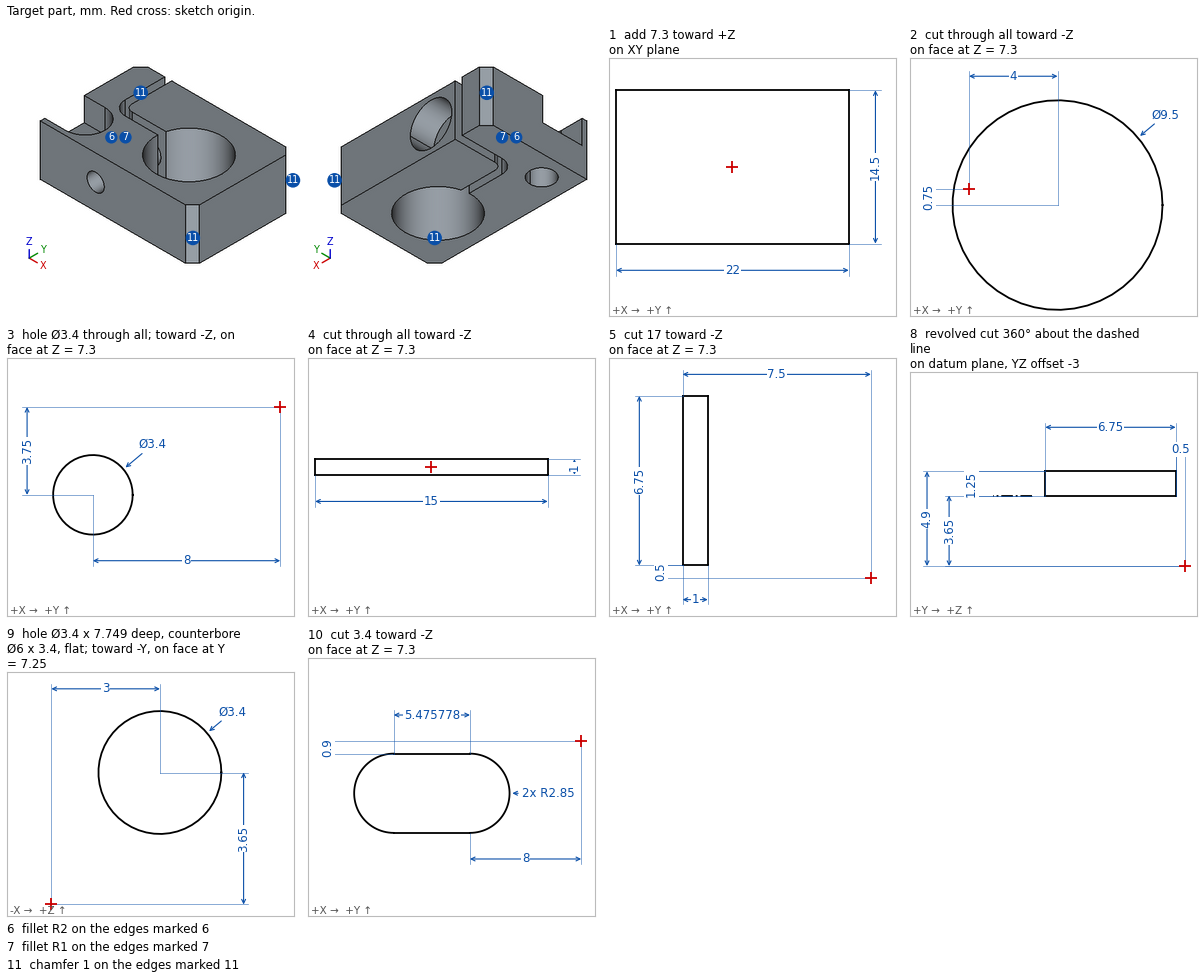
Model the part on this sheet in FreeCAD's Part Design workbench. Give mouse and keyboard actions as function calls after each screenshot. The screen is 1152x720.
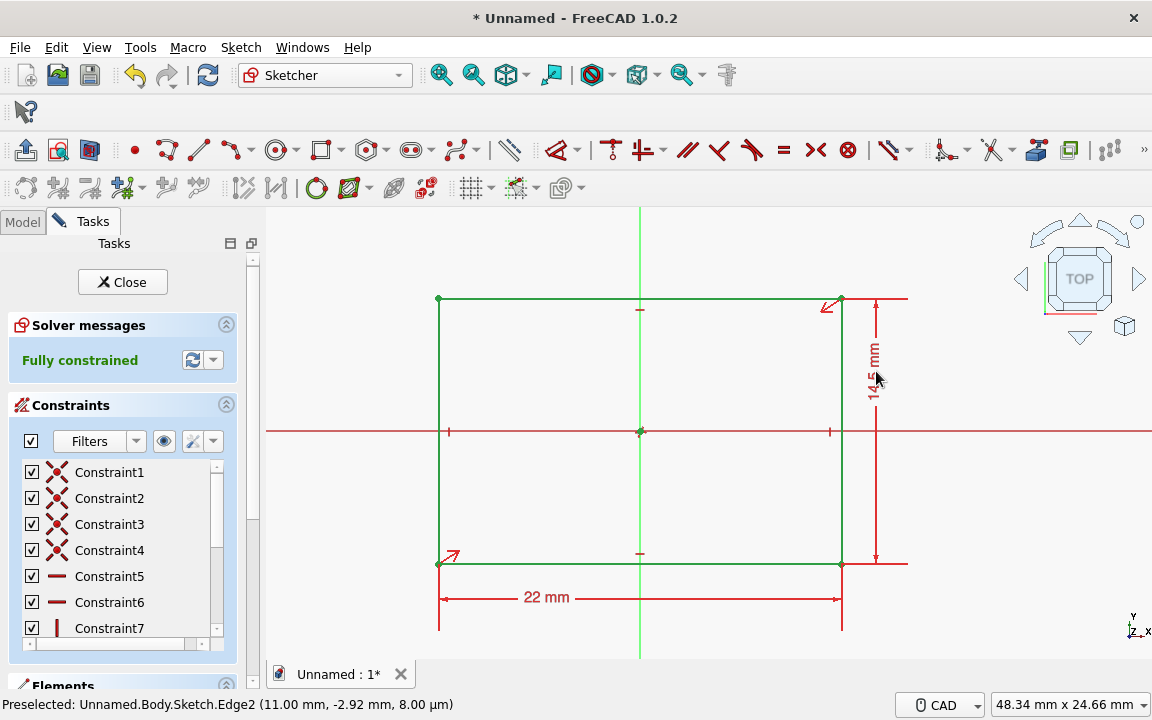
click(123, 282)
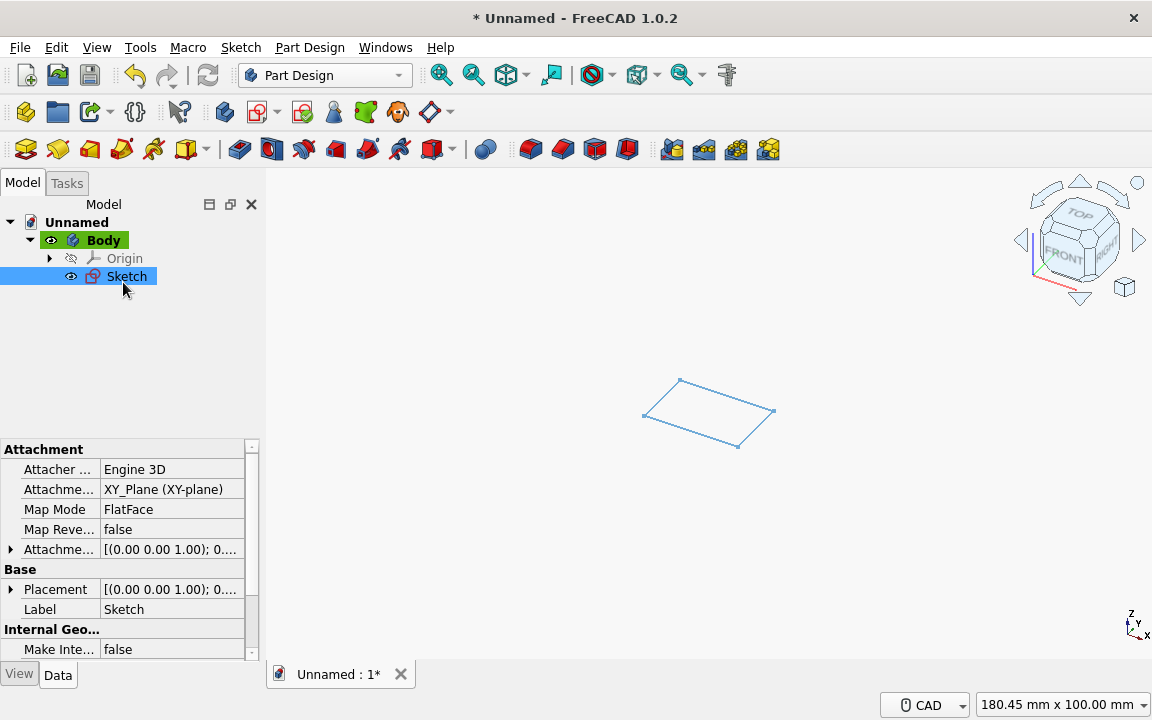
click(26, 150)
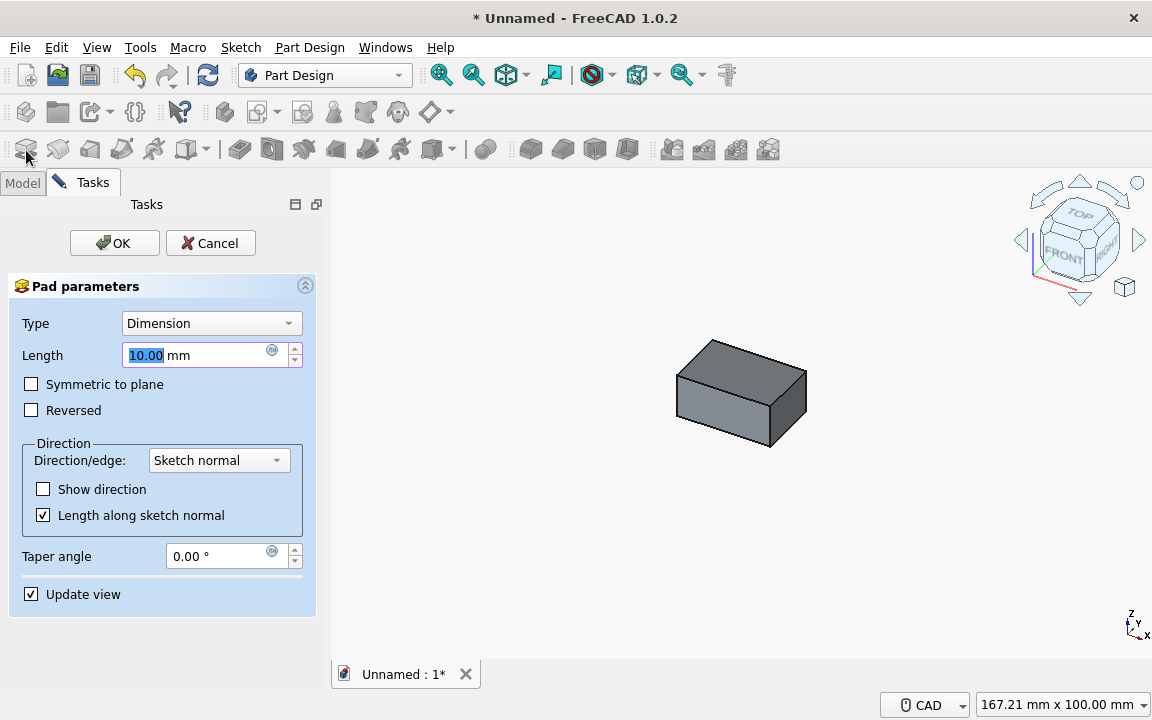
text(7.3)
key(Tab)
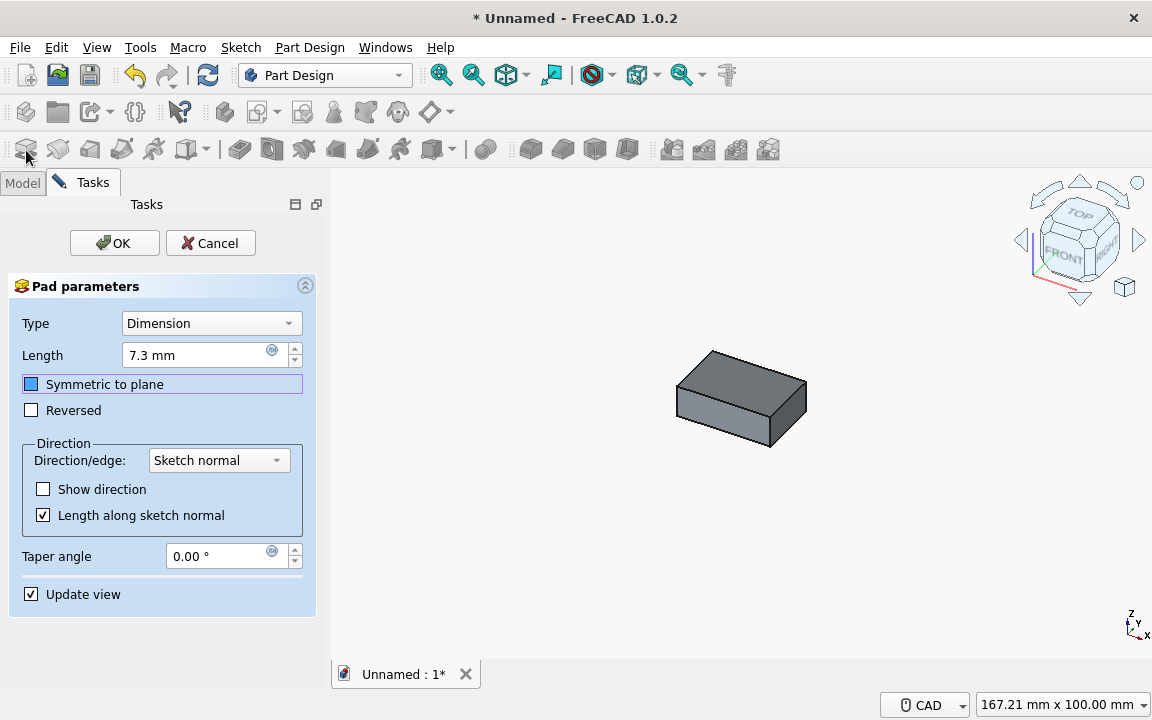
click(115, 243)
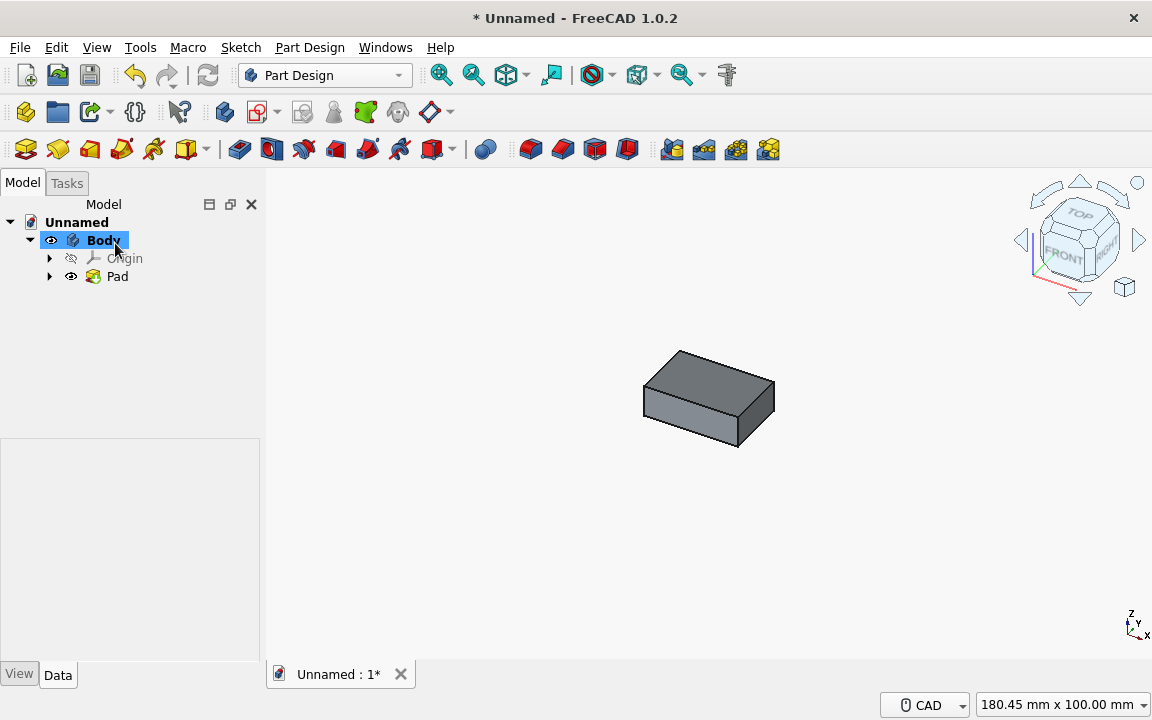
click(442, 76)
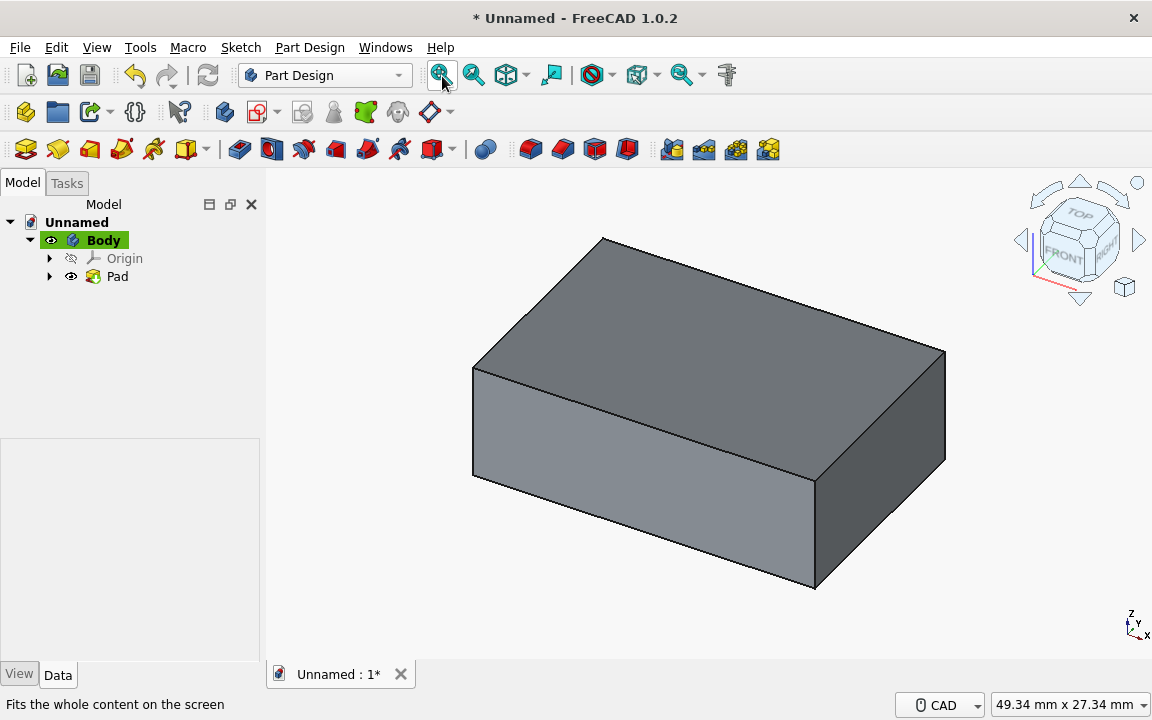
click(758, 375)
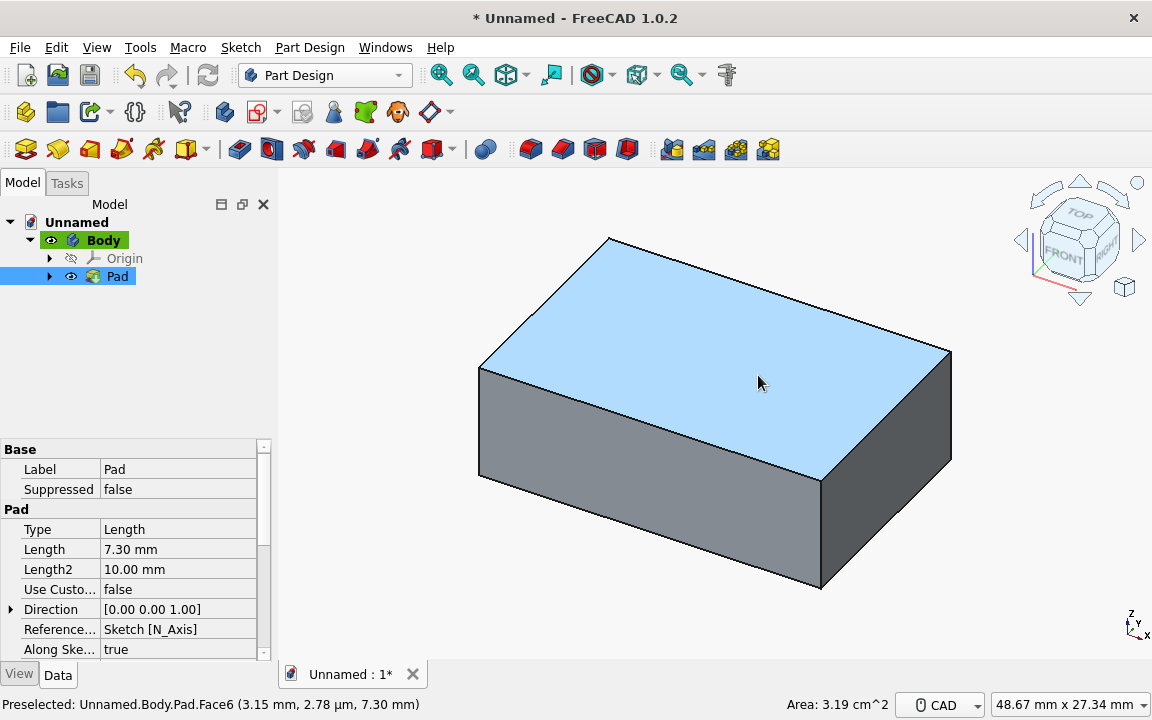
click(258, 112)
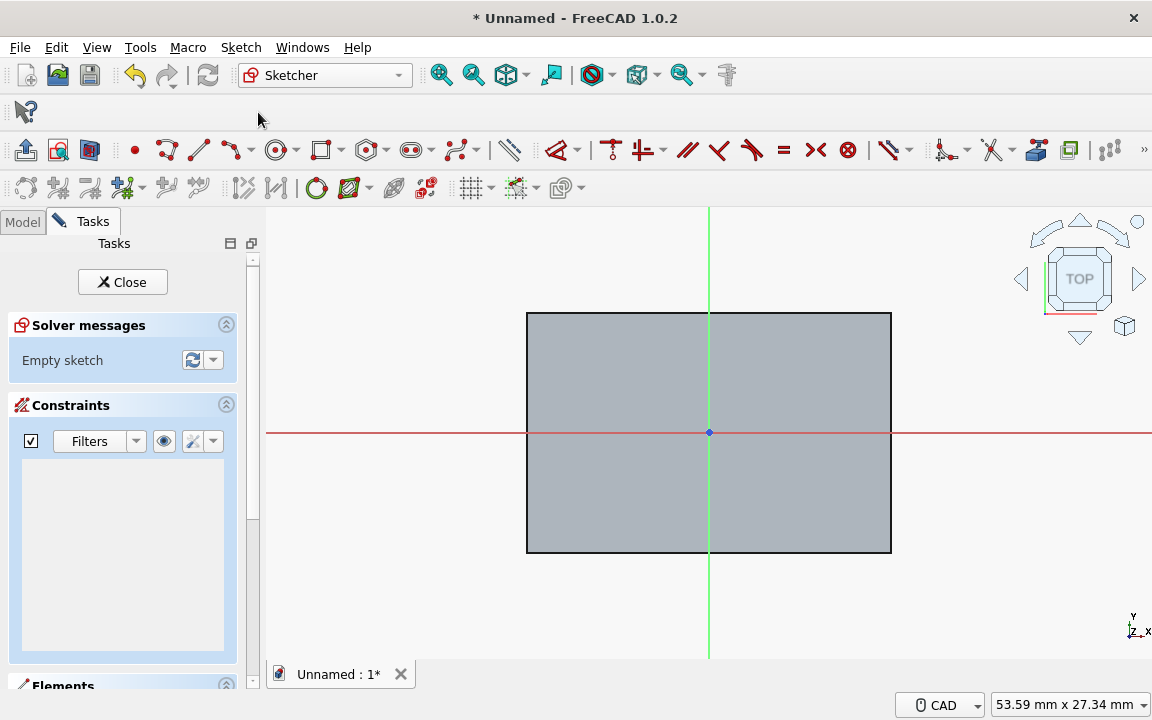
scroll(939, 460, up, 3)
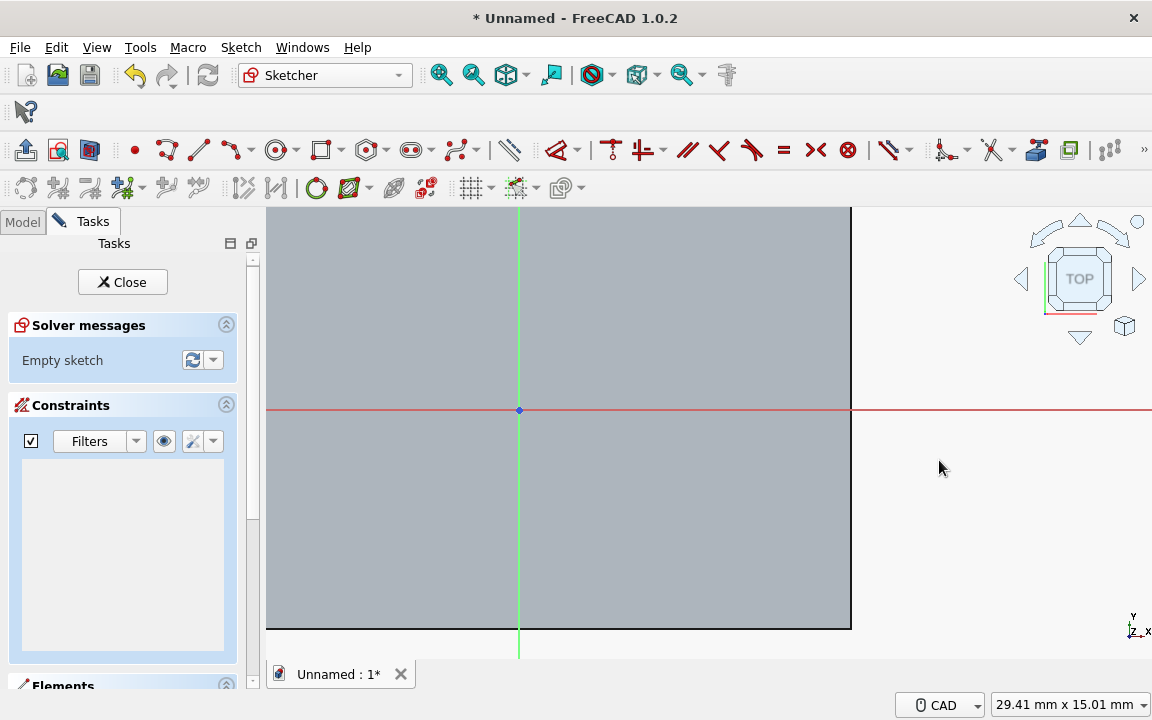
click(276, 150)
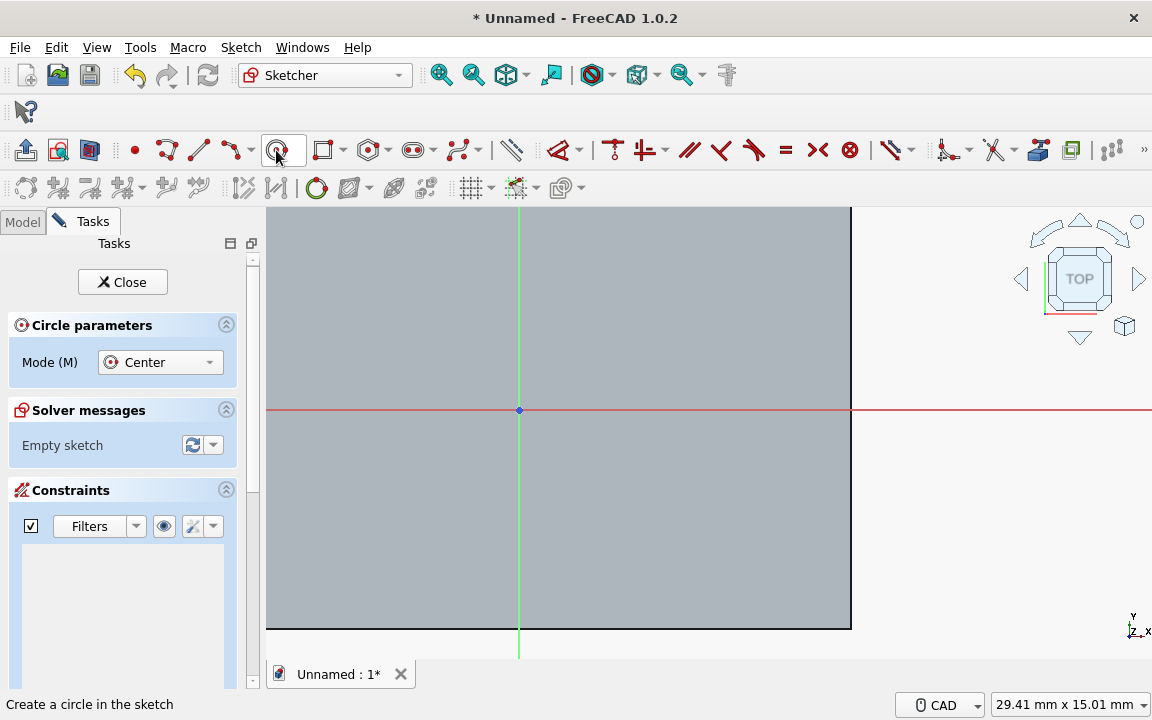
click(640, 433)
click(741, 332)
key(Escape)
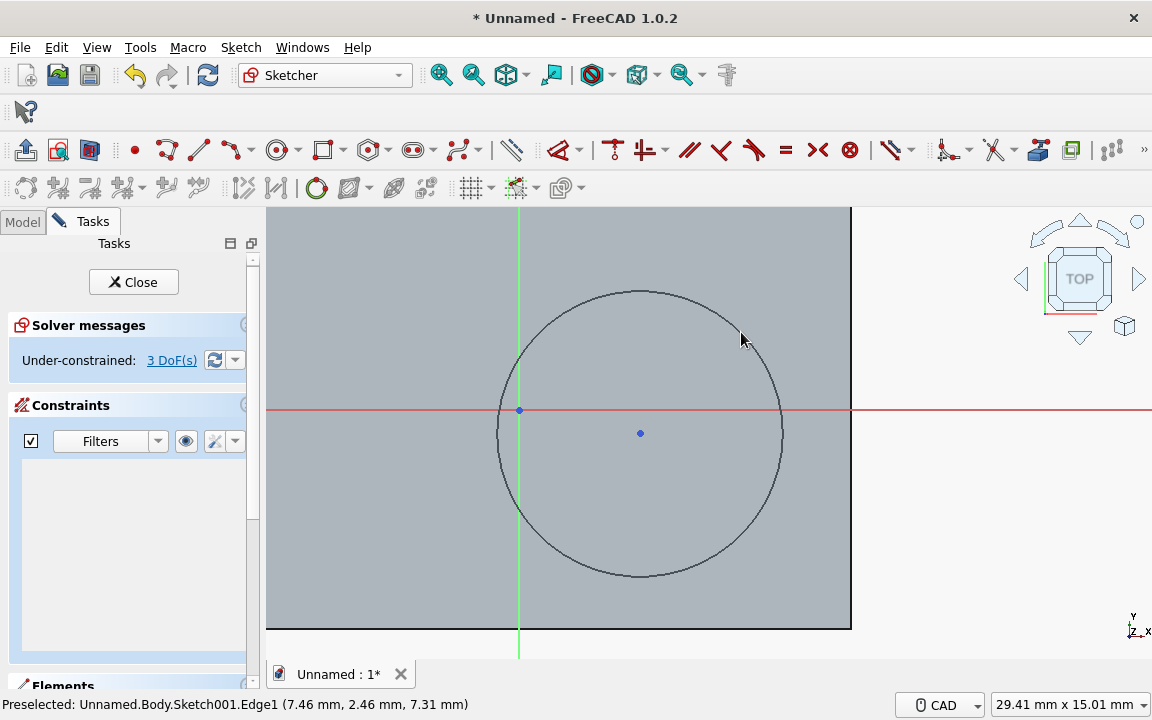
key(d)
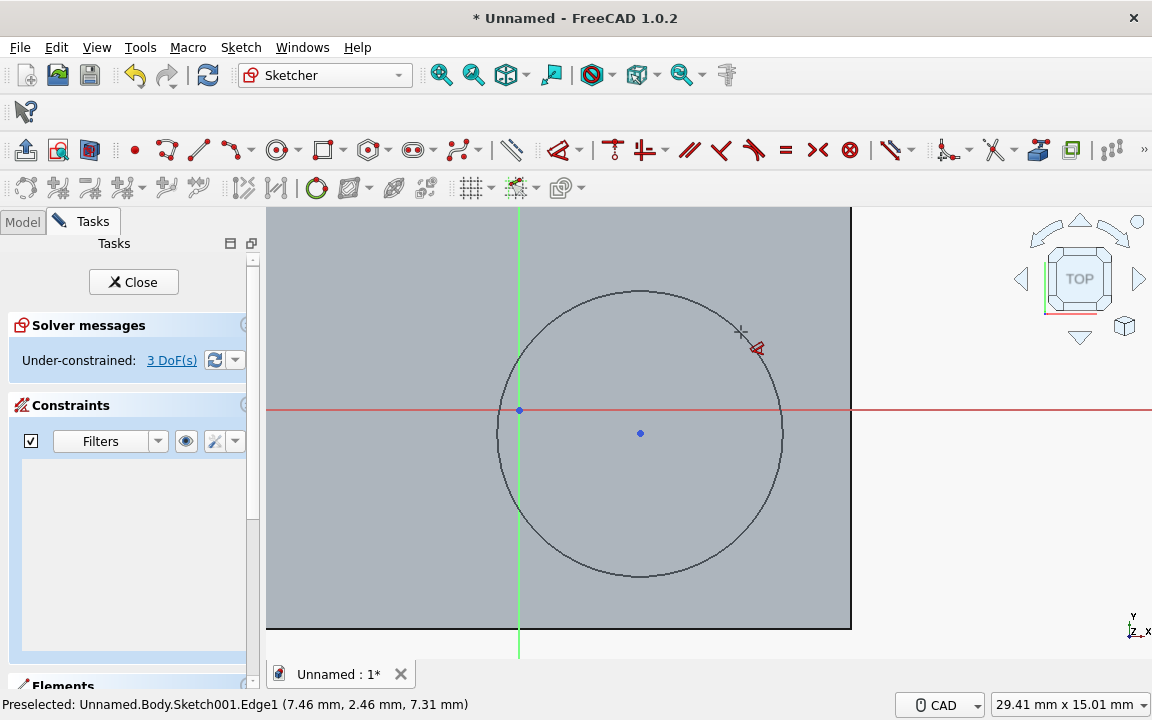
click(741, 333)
click(764, 310)